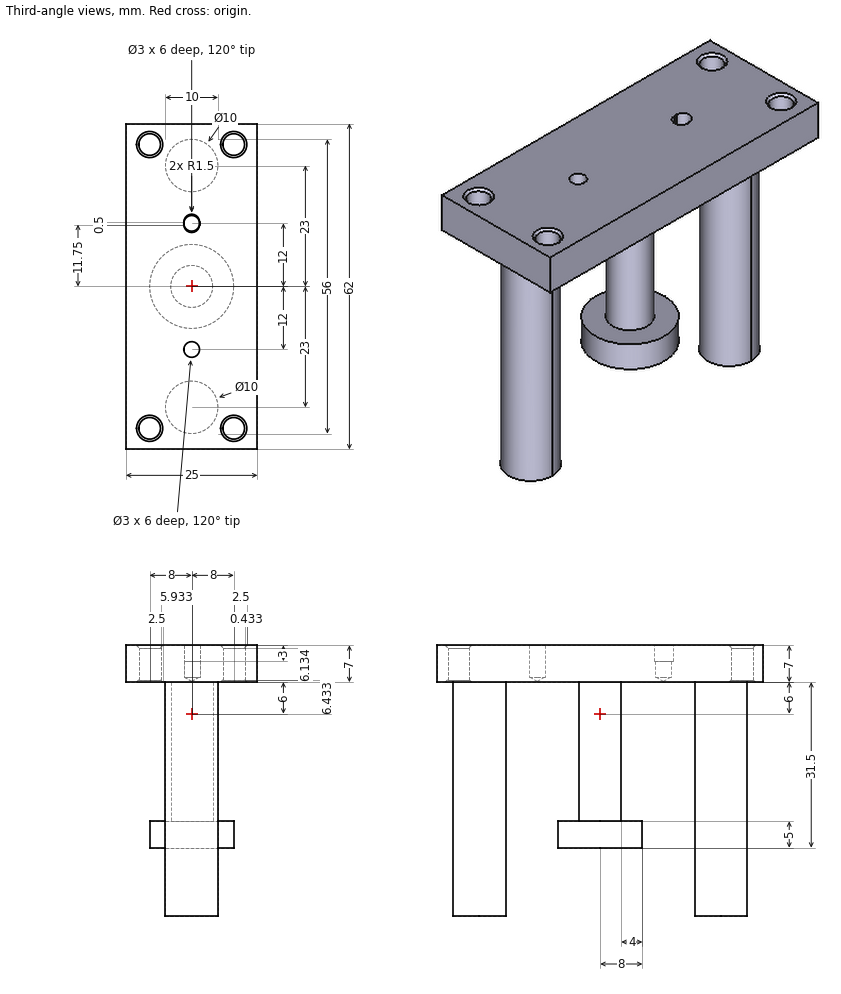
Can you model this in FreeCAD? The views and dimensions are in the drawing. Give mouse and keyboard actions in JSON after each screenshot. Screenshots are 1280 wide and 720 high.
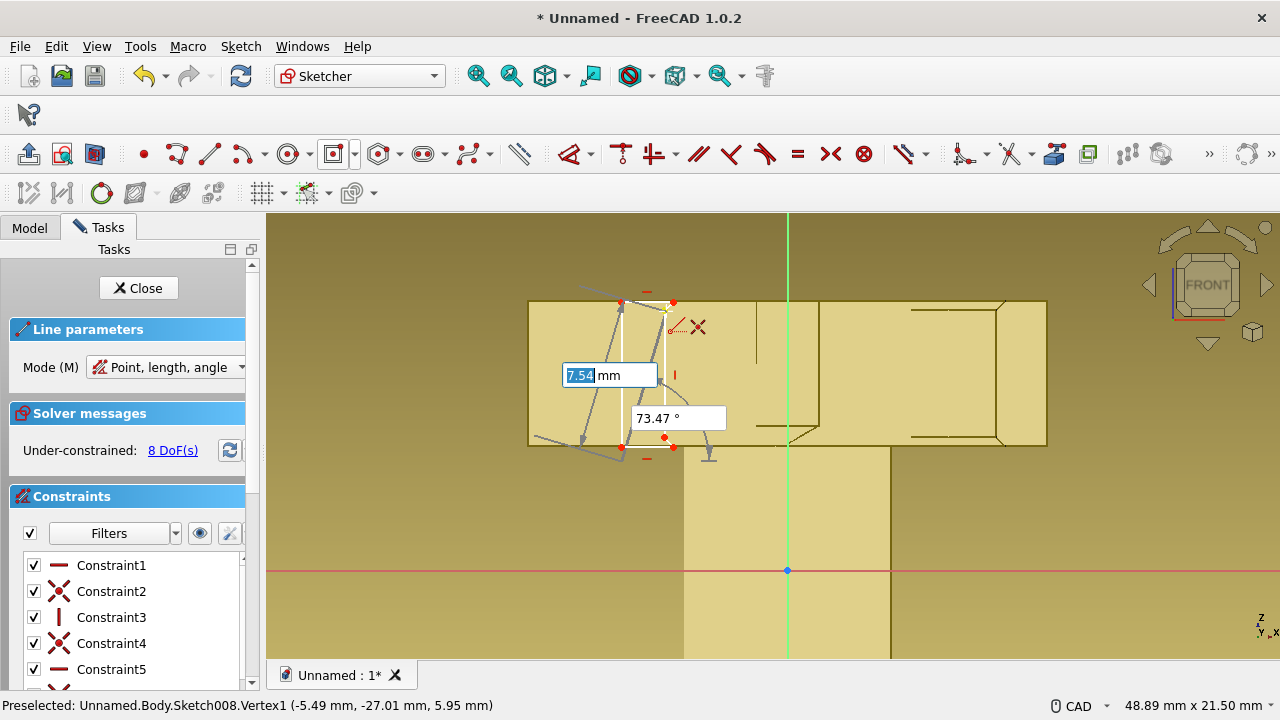
{"action": "left_click", "coordinate": [622, 505]}
{"action": "key", "text": "Escape"}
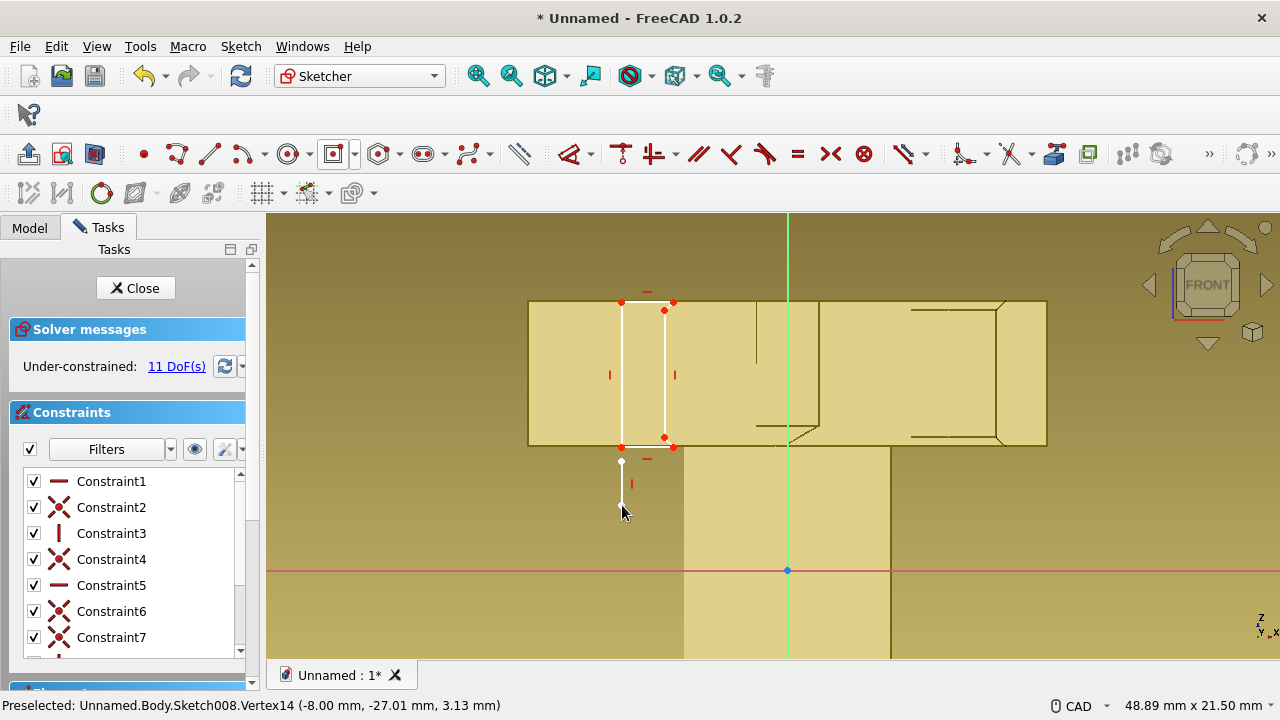
{"action": "left_click", "coordinate": [622, 475]}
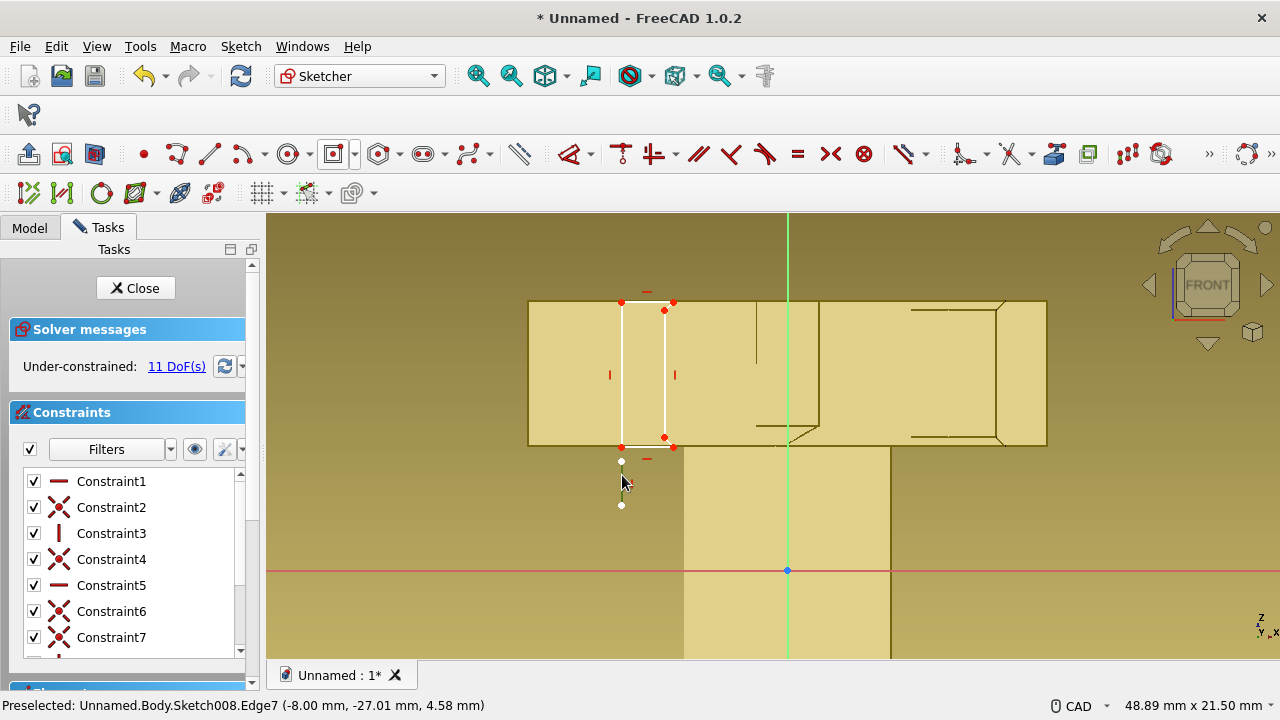
{"action": "left_click", "coordinate": [520, 154]}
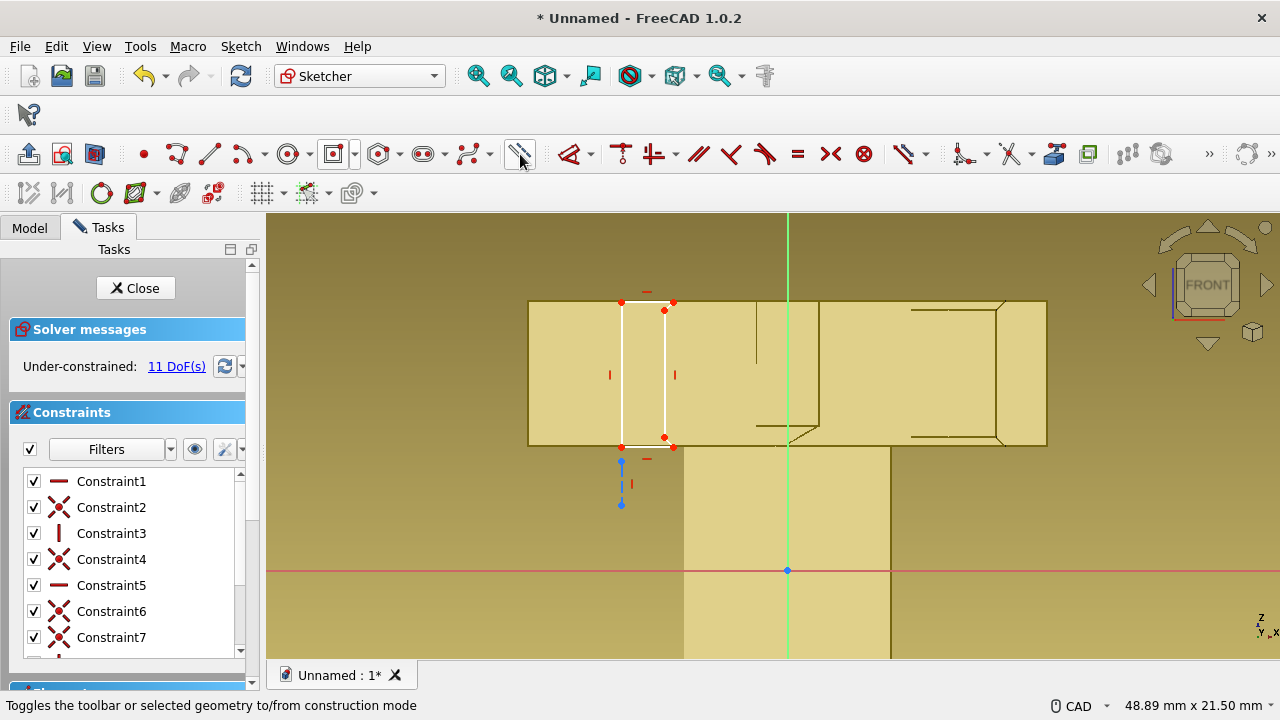
{"action": "left_click", "coordinate": [568, 154]}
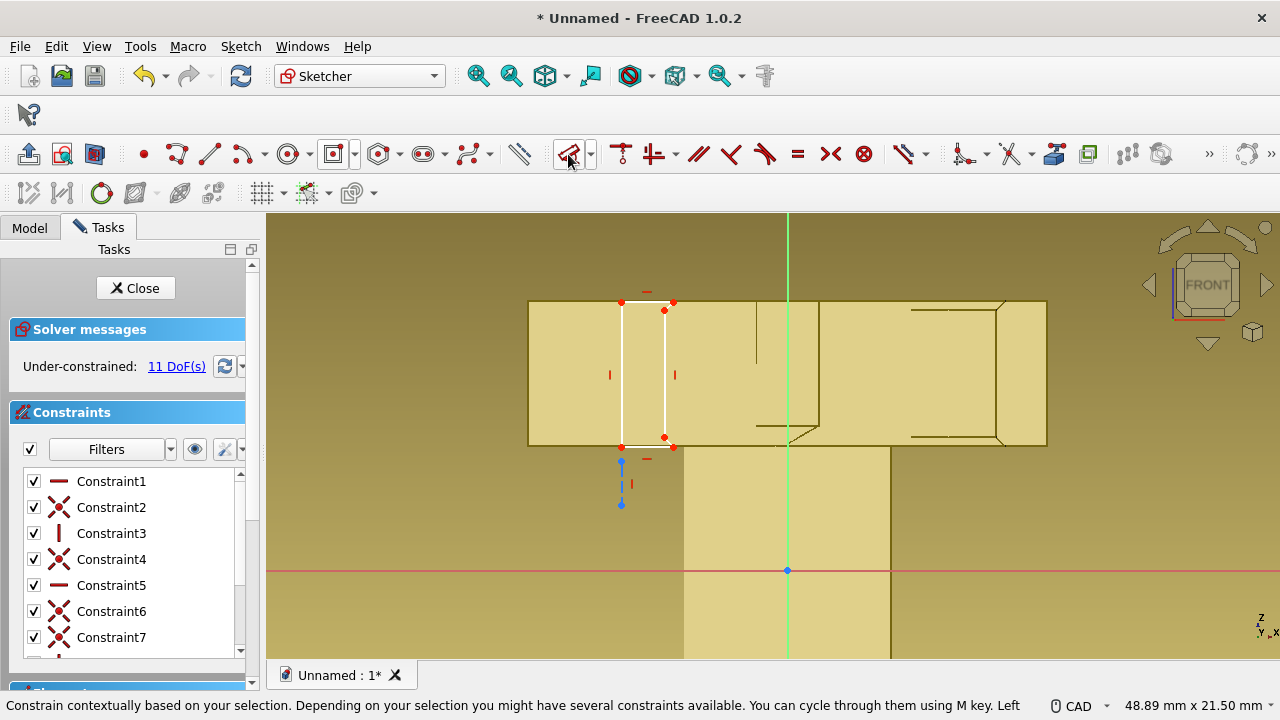
{"action": "left_click", "coordinate": [622, 404]}
{"action": "left_click", "coordinate": [588, 375]}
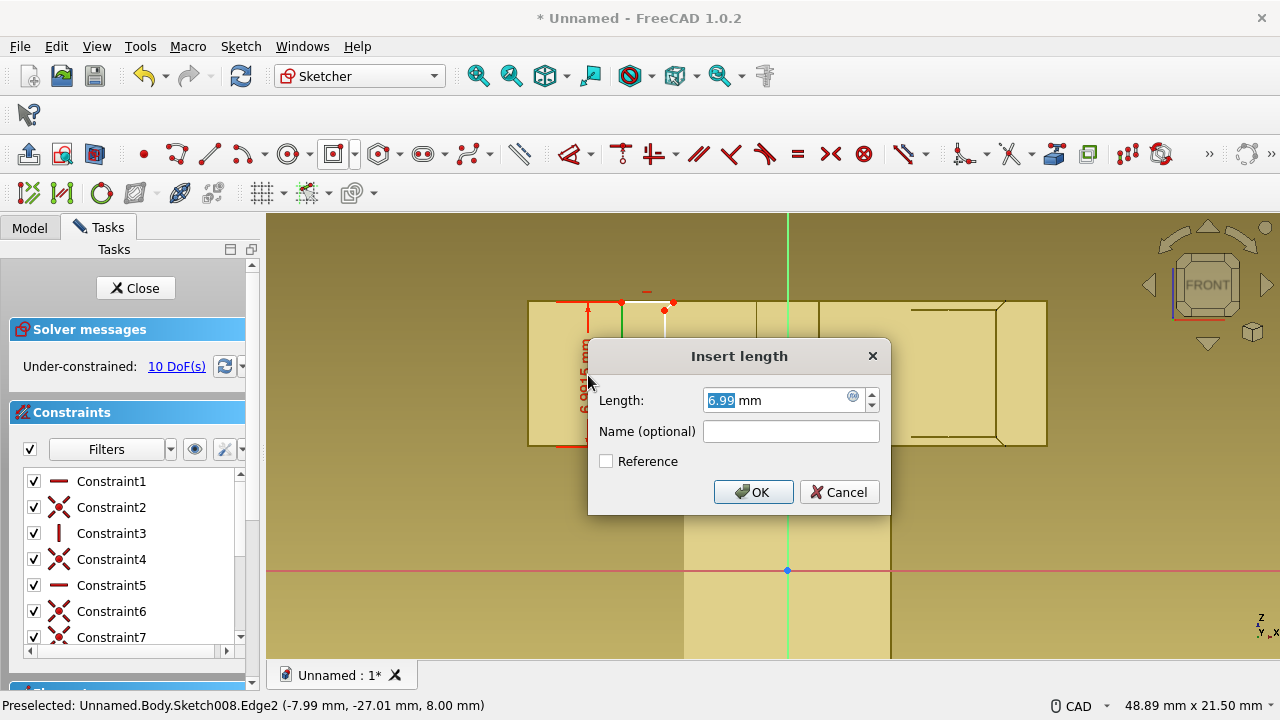
{"action": "type", "text": "7"}
{"action": "key", "text": "Return"}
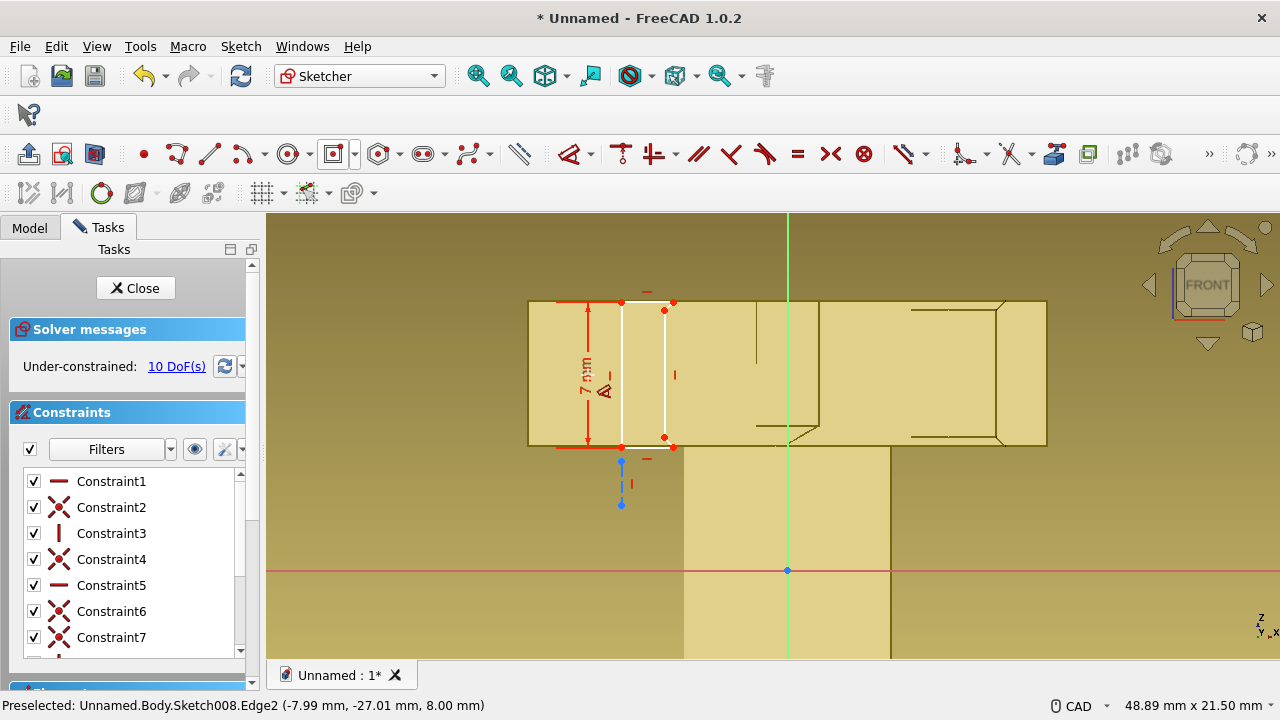
{"action": "left_click", "coordinate": [674, 448]}
{"action": "left_click", "coordinate": [822, 509]}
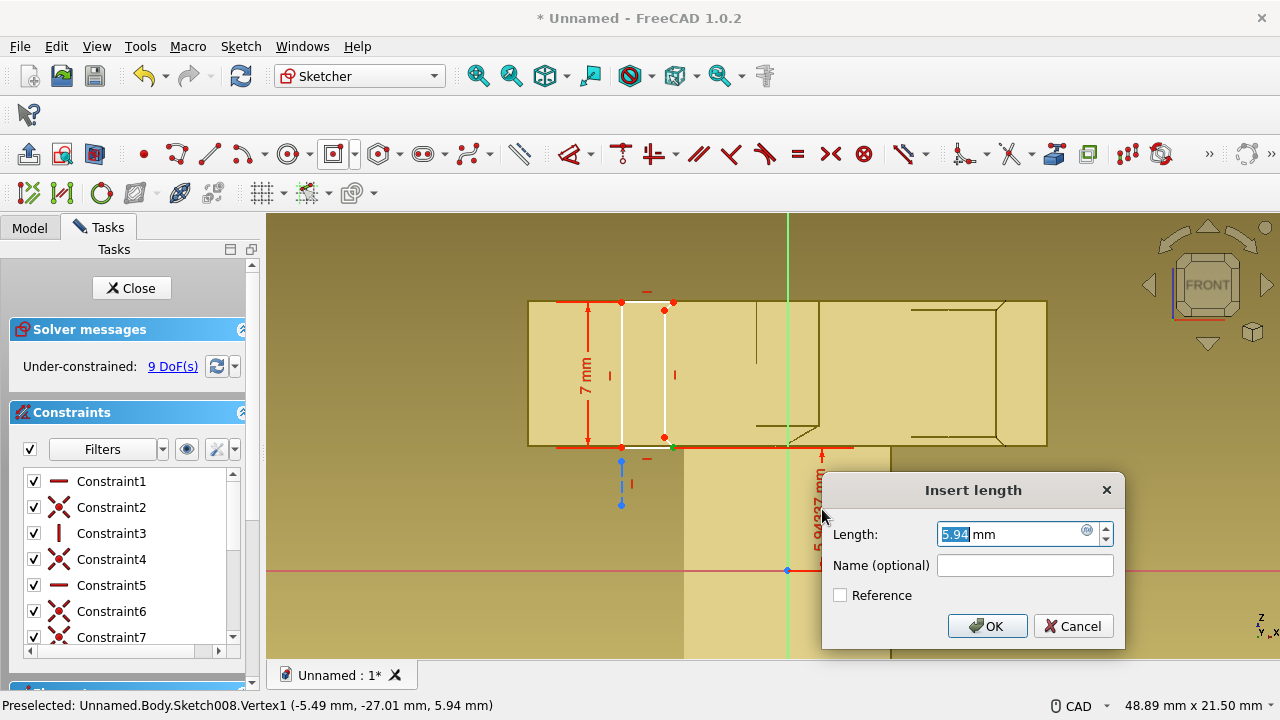
{"action": "type", "text": "6"}
{"action": "key", "text": "Return"}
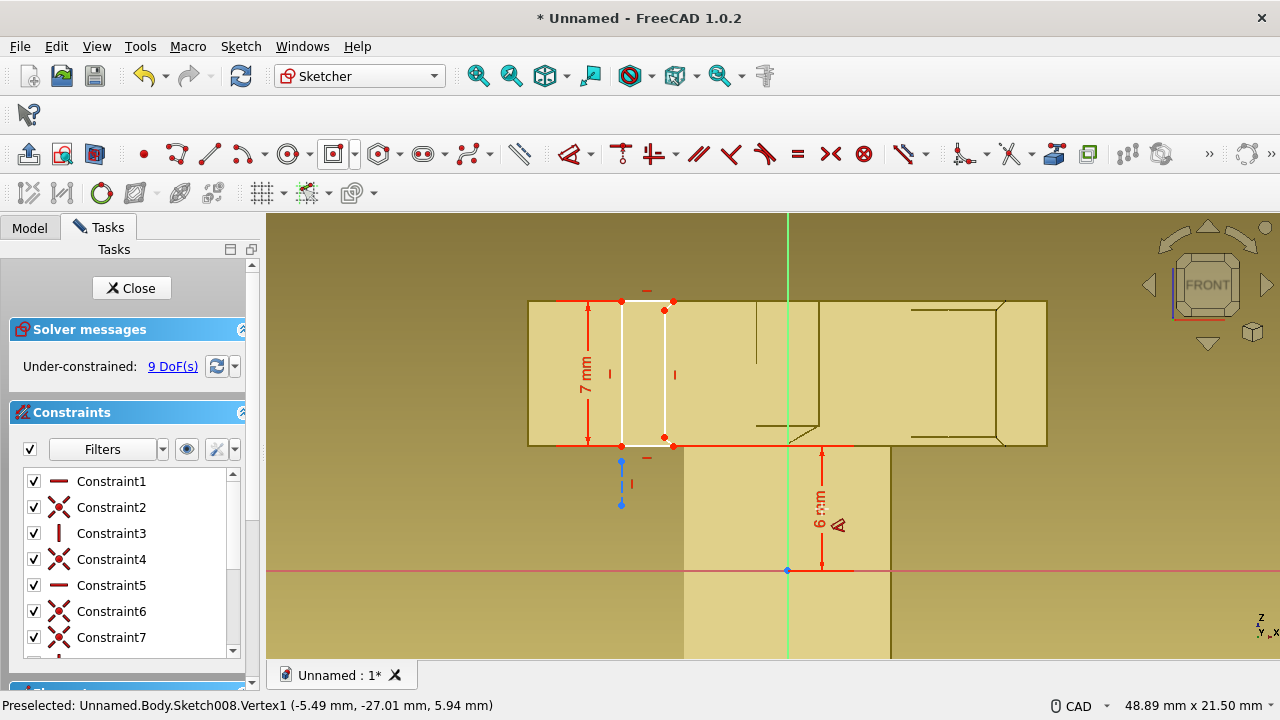
{"action": "left_click", "coordinate": [622, 446]}
{"action": "left_click", "coordinate": [705, 605]}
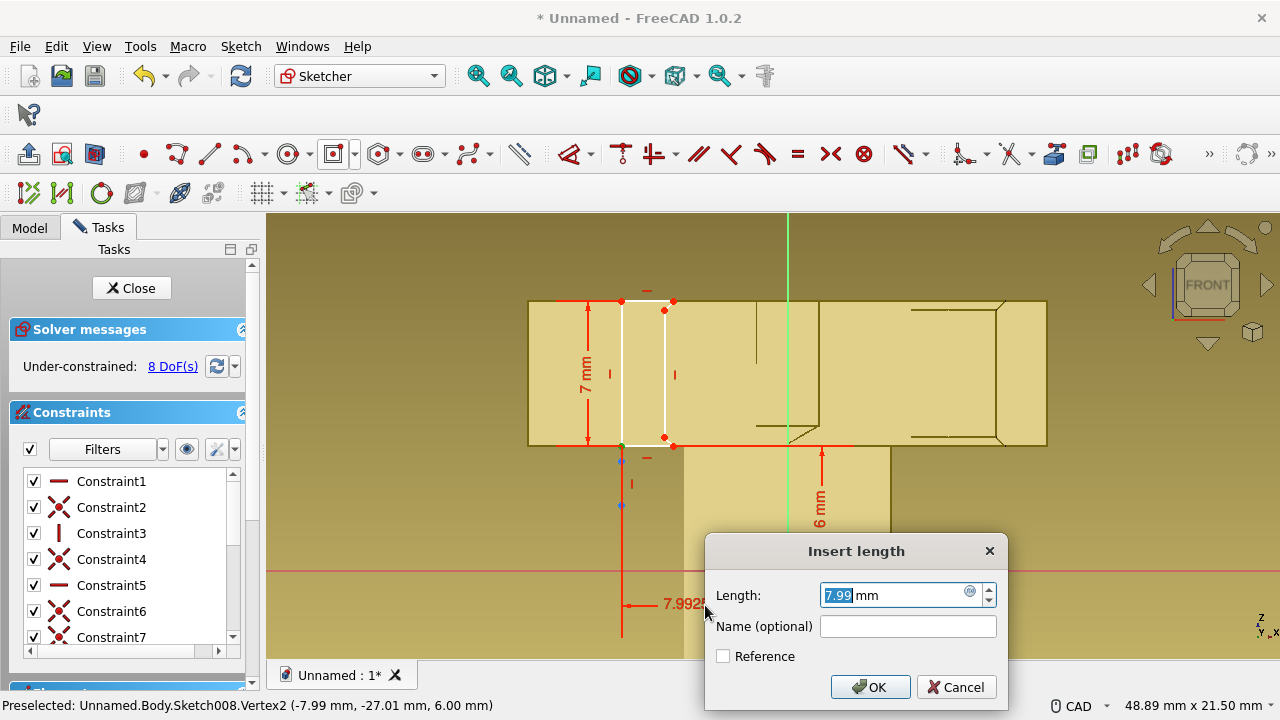
{"action": "type", "text": "8"}
{"action": "key", "text": "Return"}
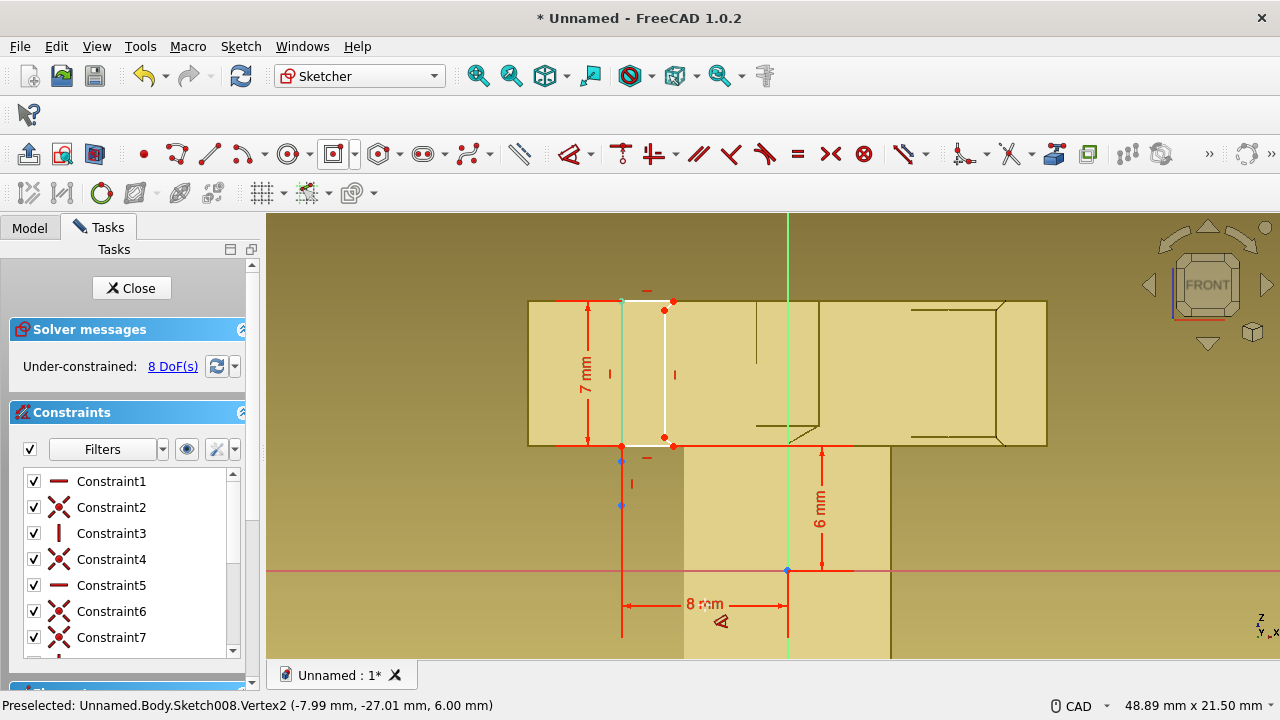
{"action": "left_click", "coordinate": [622, 461]}
{"action": "left_click", "coordinate": [705, 427]}